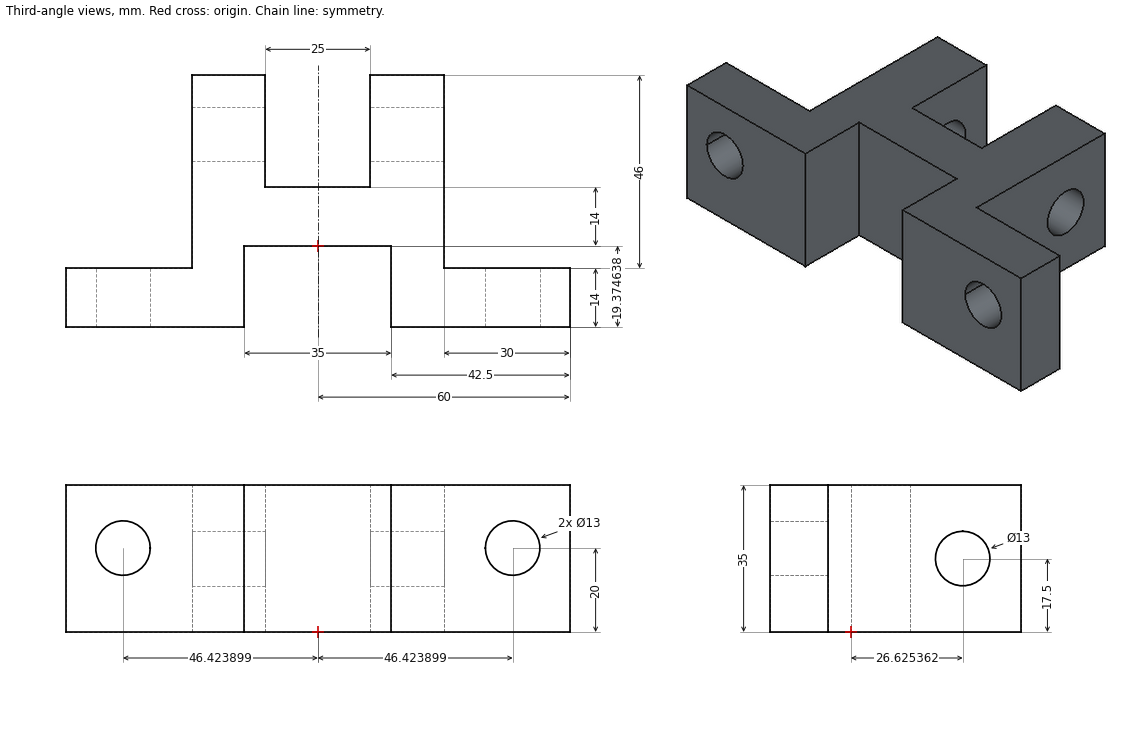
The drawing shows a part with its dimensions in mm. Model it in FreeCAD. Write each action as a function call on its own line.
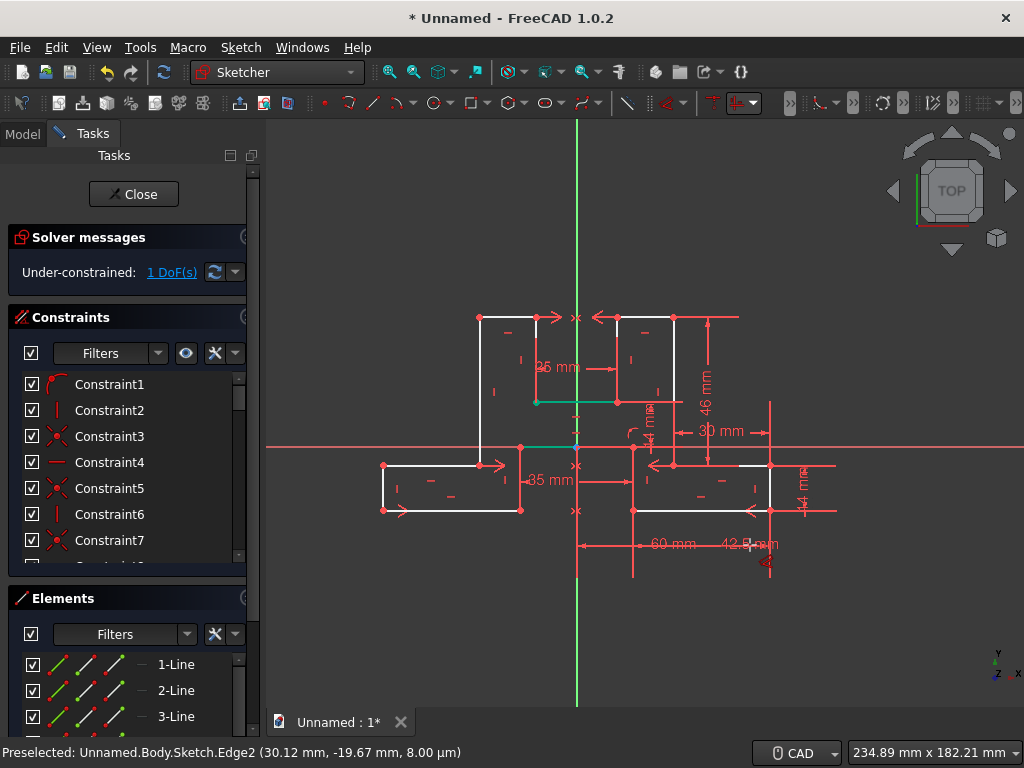
click(633, 466)
click(667, 479)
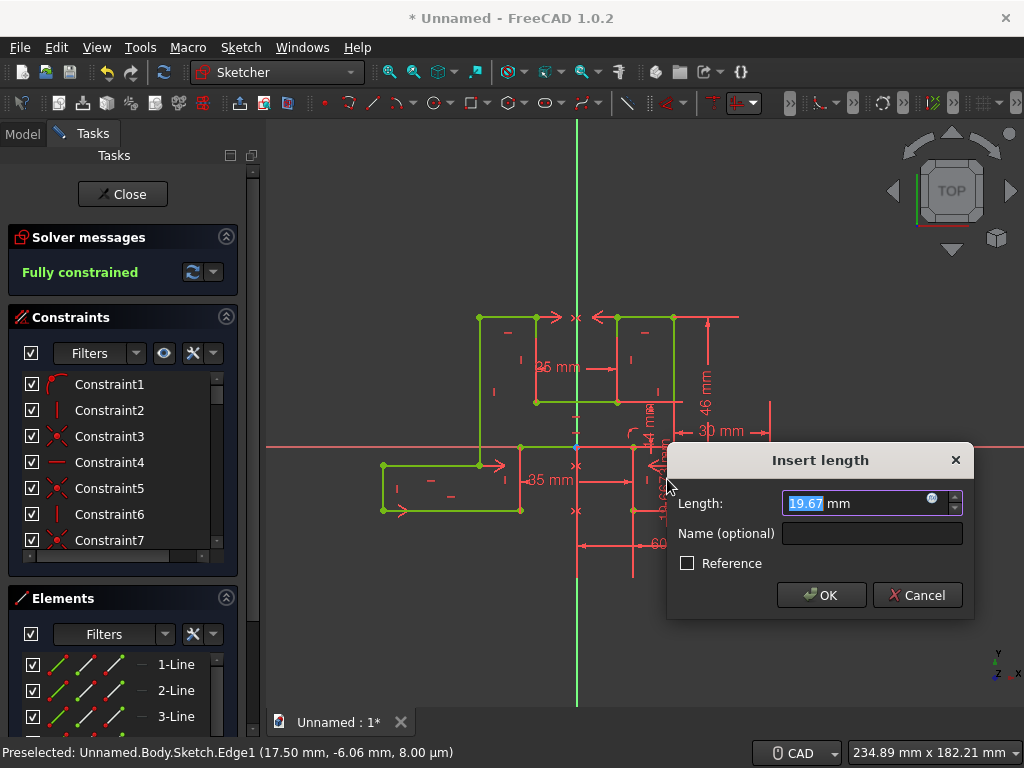
text(19.374638)
key(Return)
key(Escape)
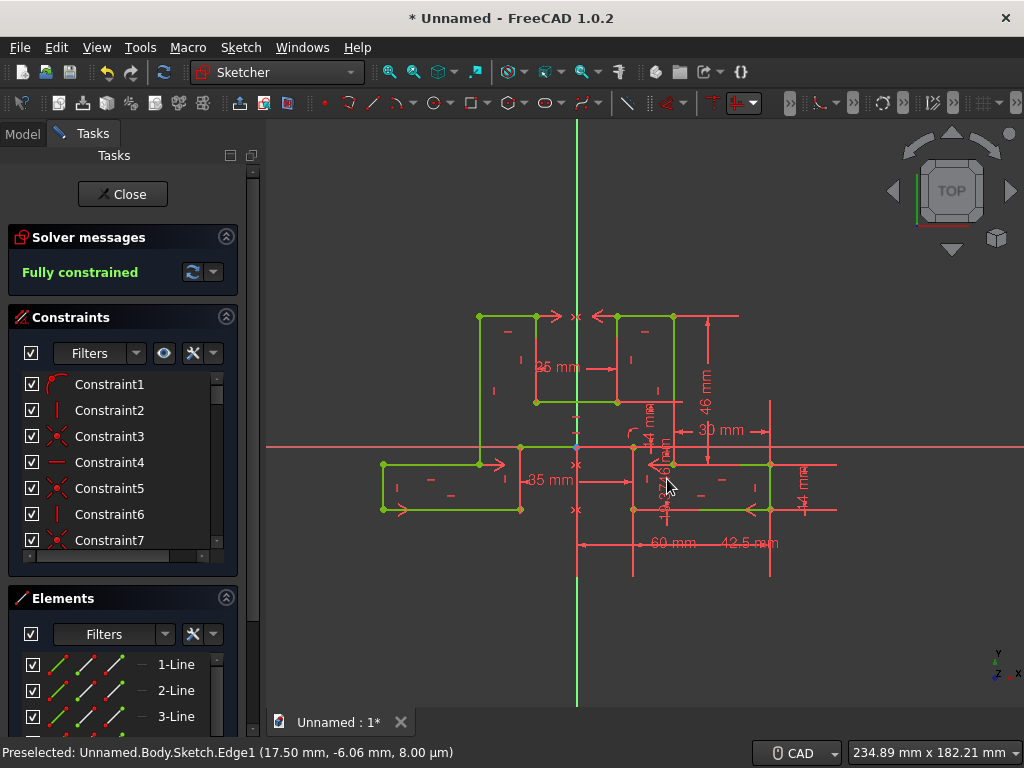
click(123, 194)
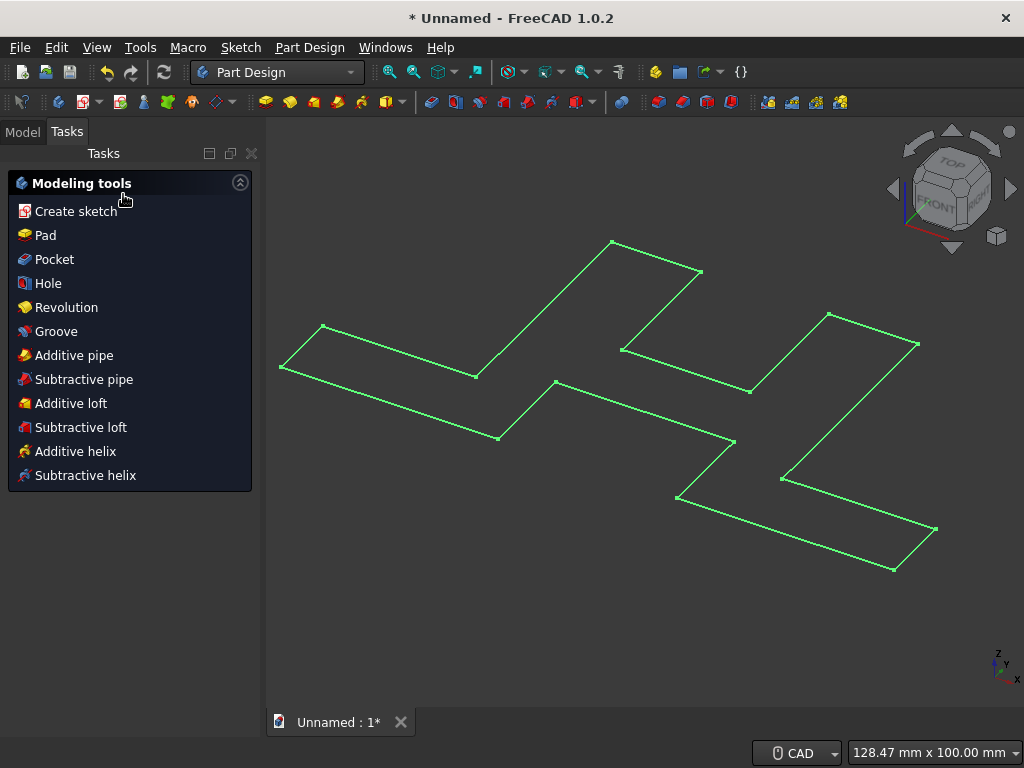
click(266, 102)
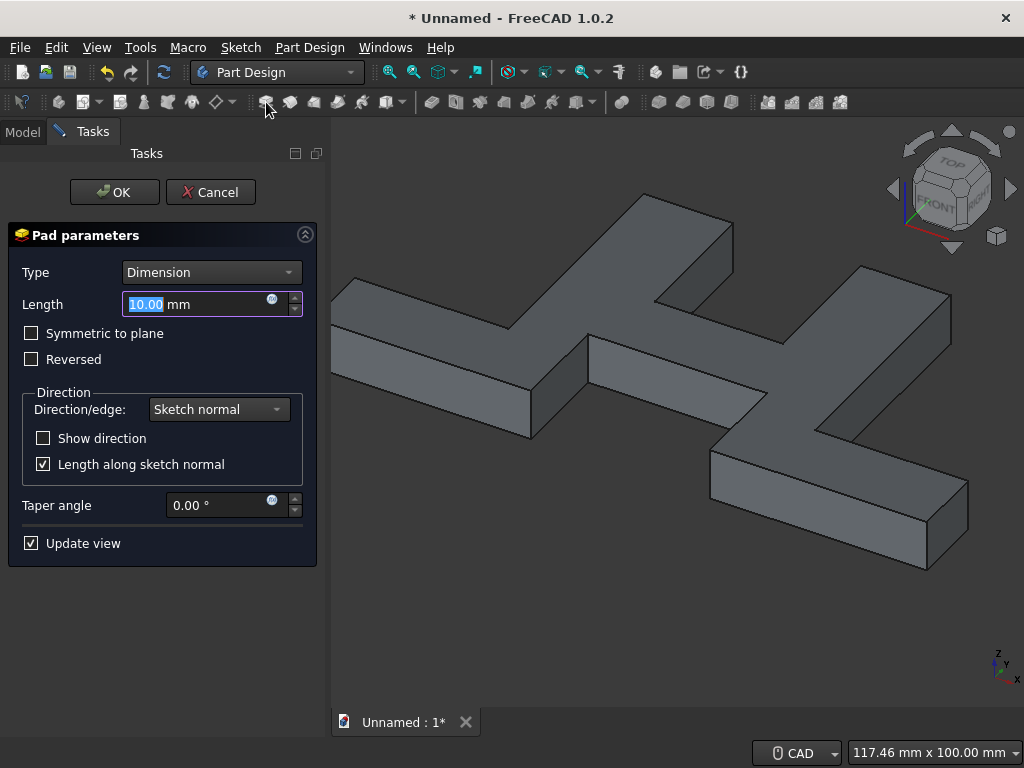
text(35)
key(Tab)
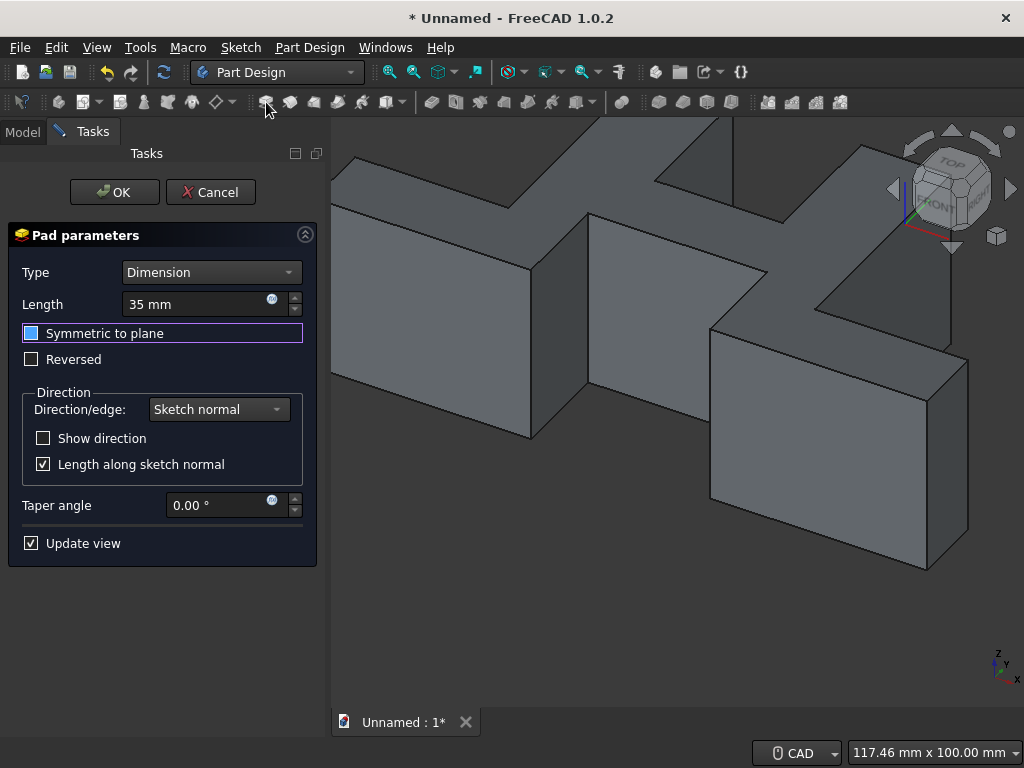
click(115, 192)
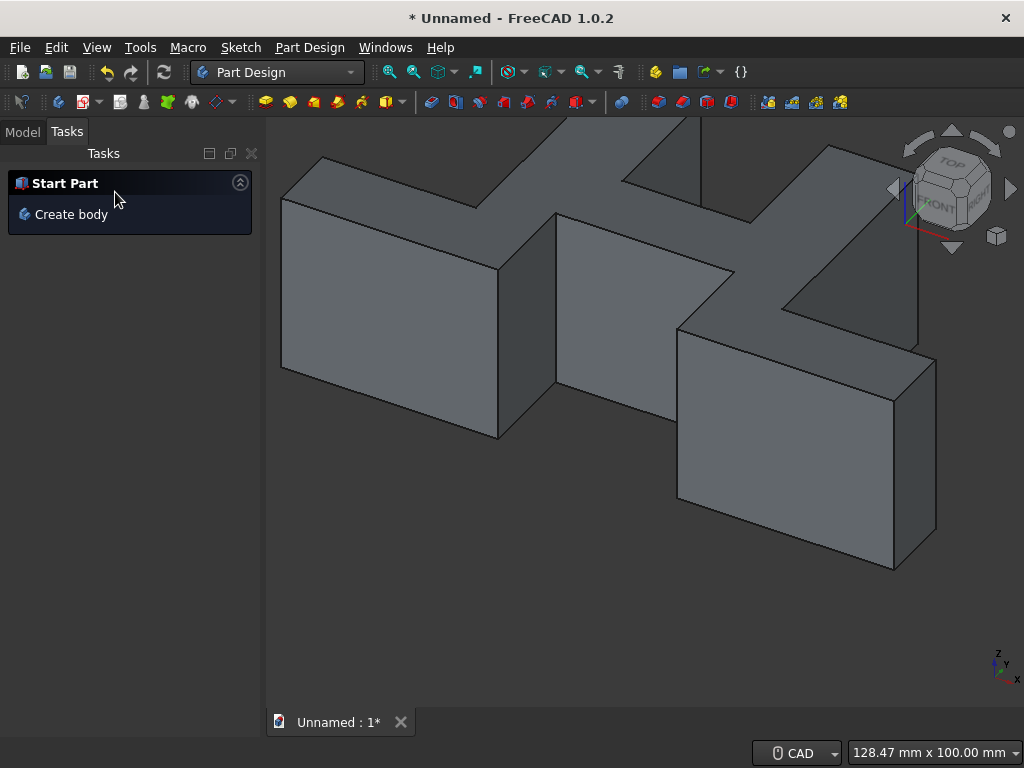
click(390, 72)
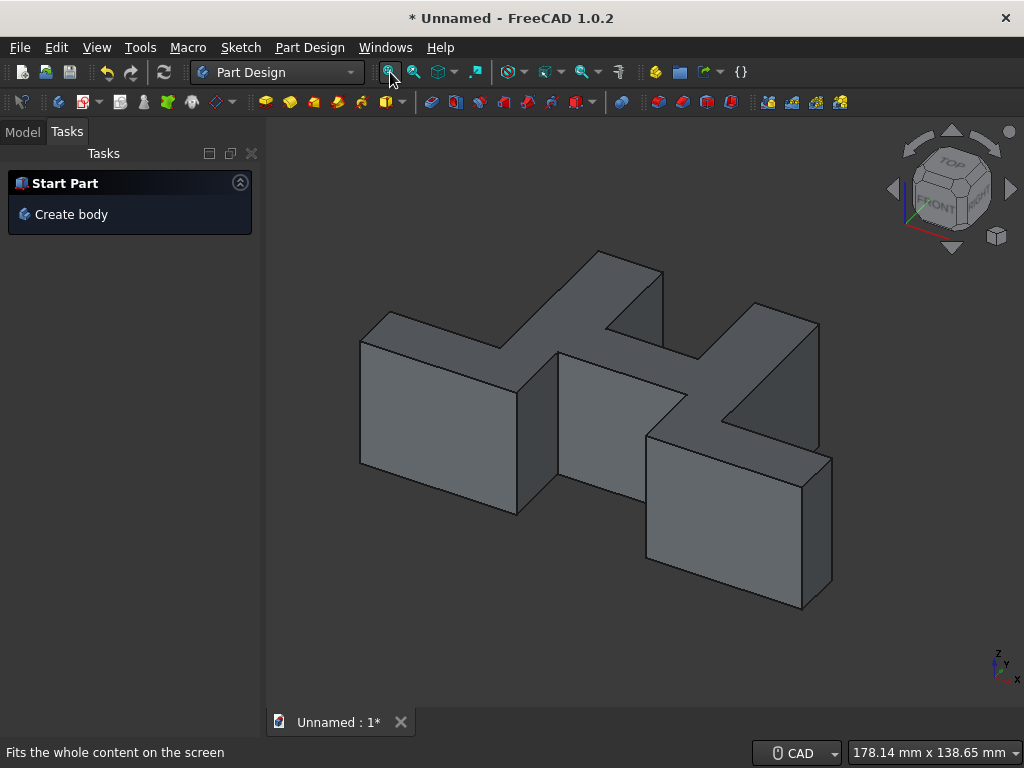
key(6)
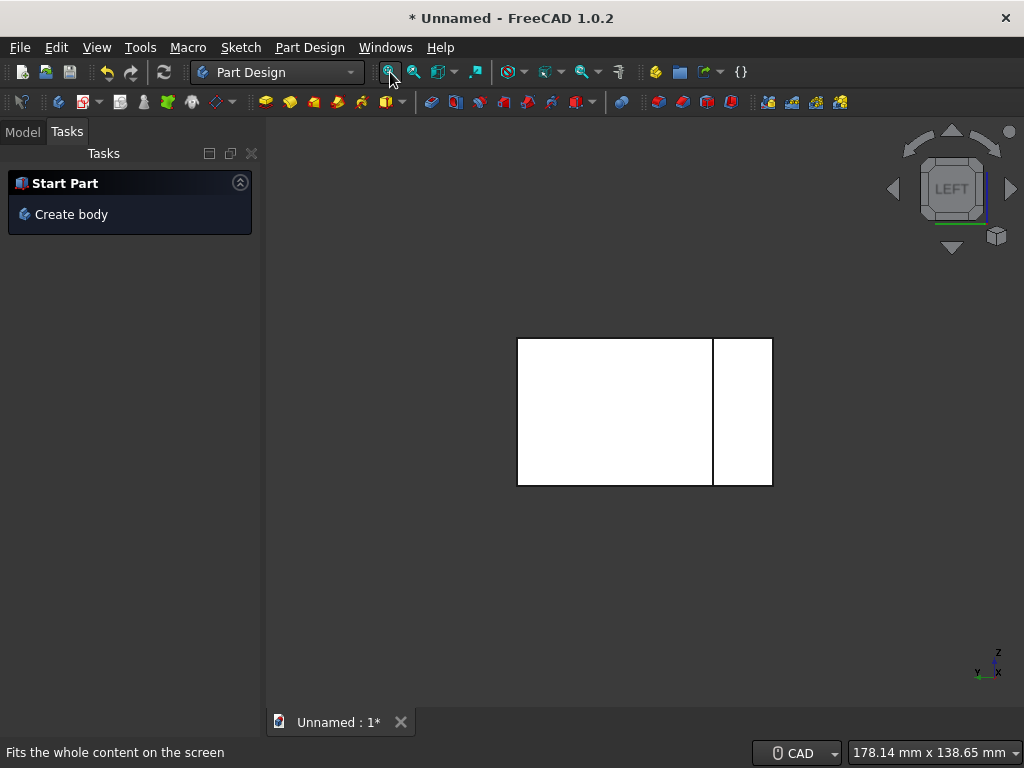
click(390, 72)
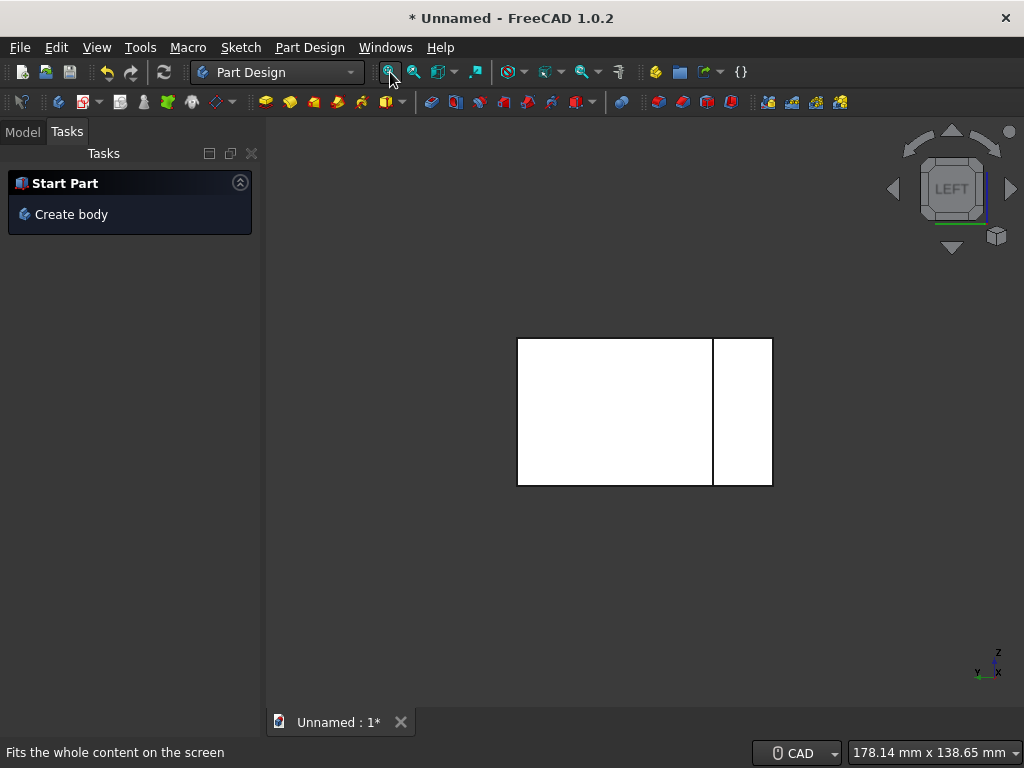
click(615, 411)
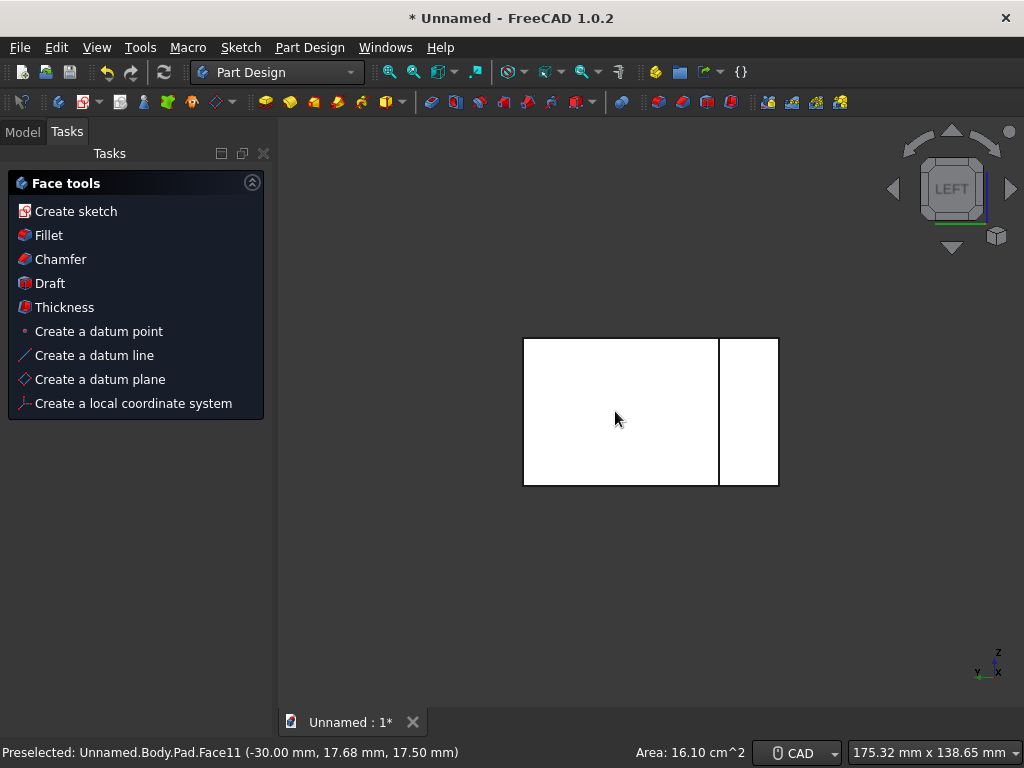
click(84, 102)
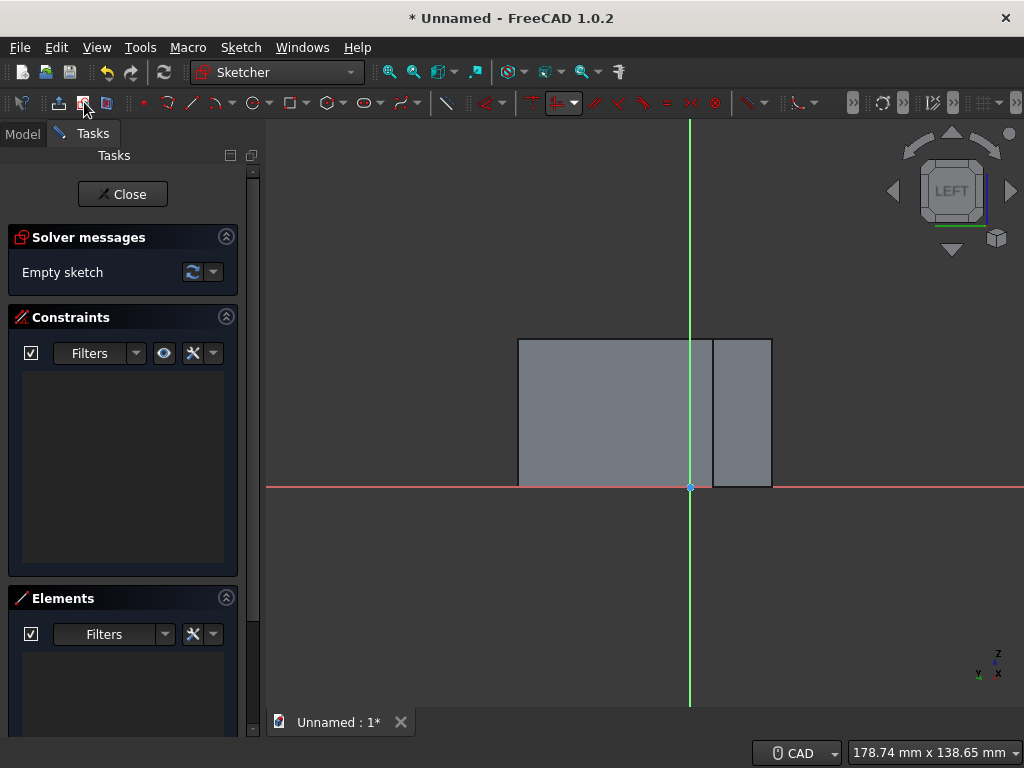
click(108, 104)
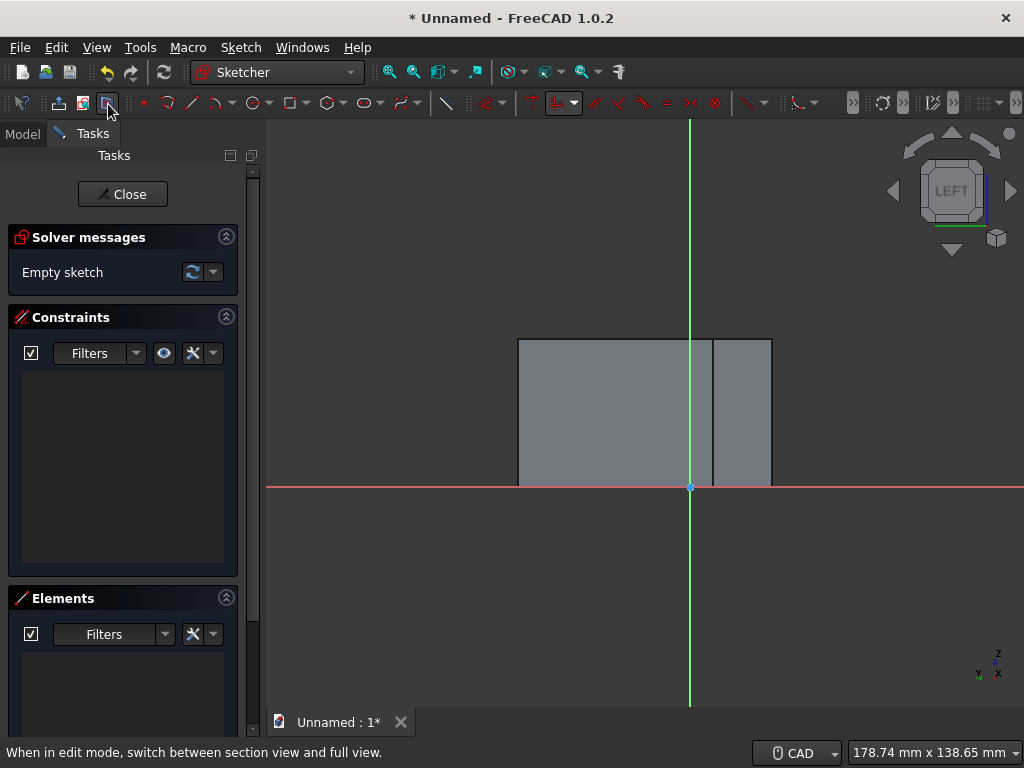
scroll(577, 413, up, 10)